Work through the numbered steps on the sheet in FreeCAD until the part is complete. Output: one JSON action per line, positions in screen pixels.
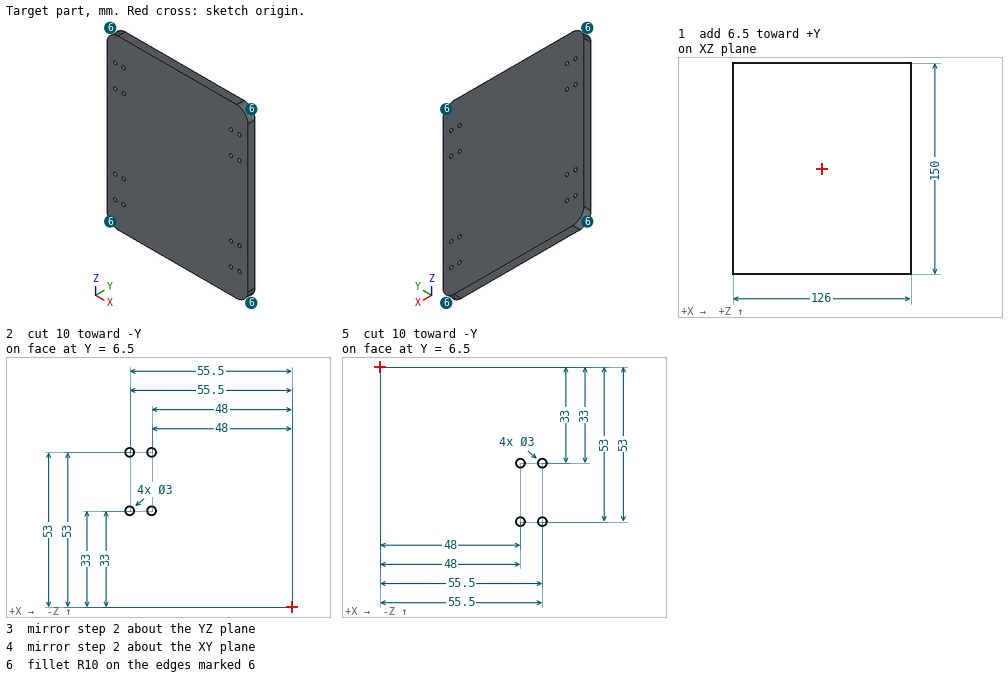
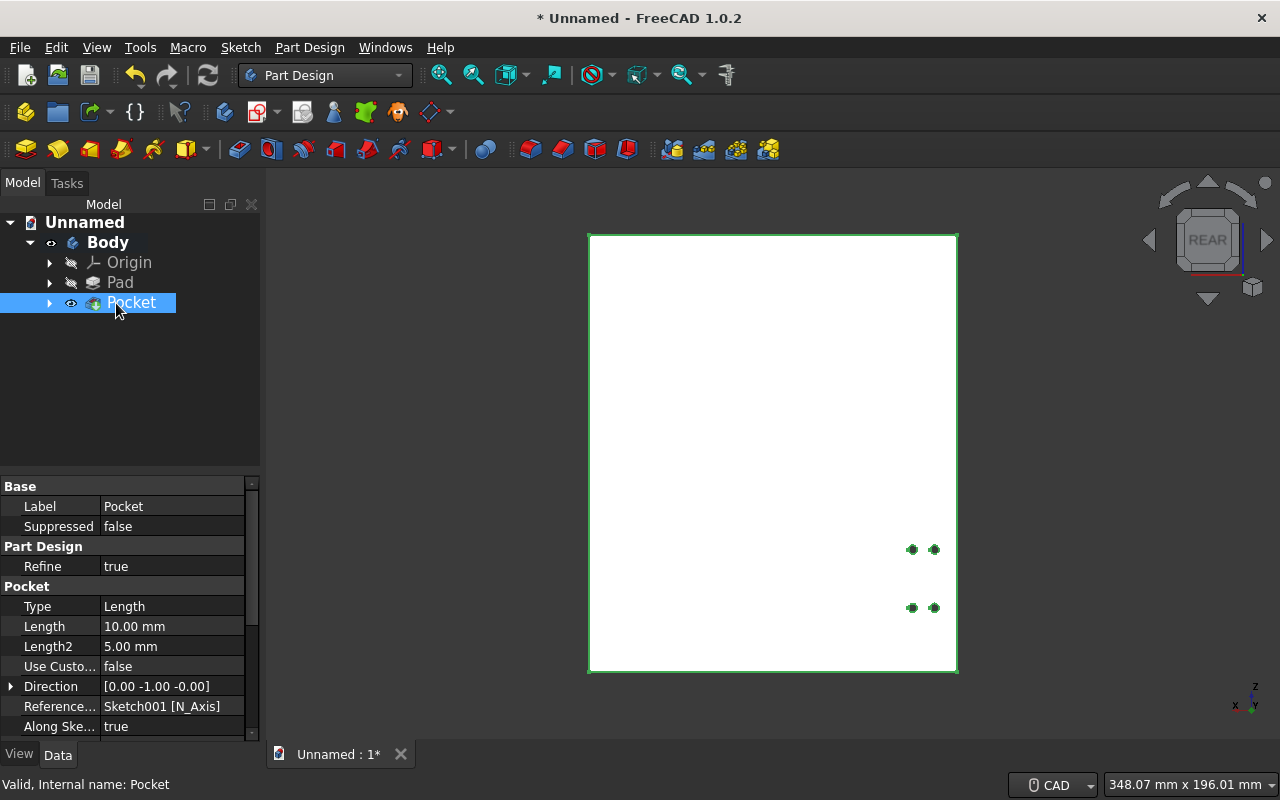
{"action": "left_click", "coordinate": [672, 150]}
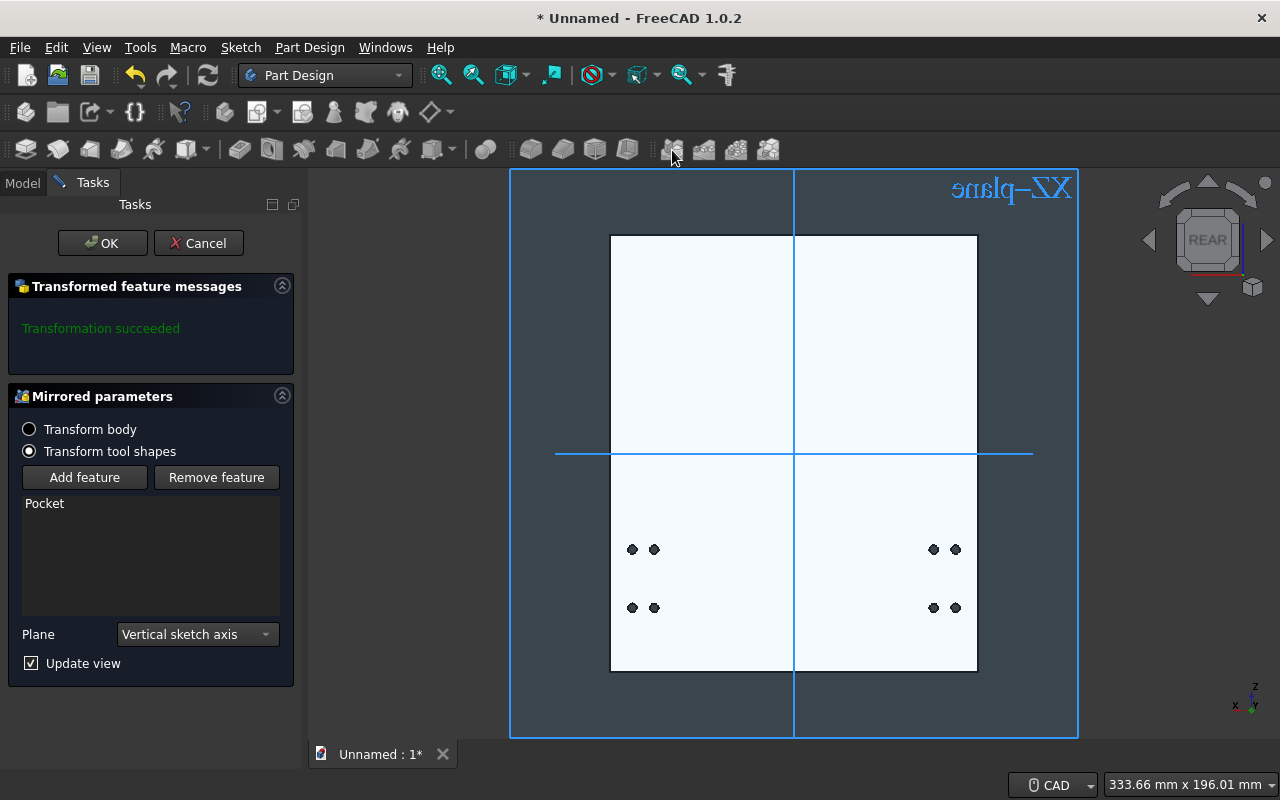
{"action": "left_click", "coordinate": [198, 634]}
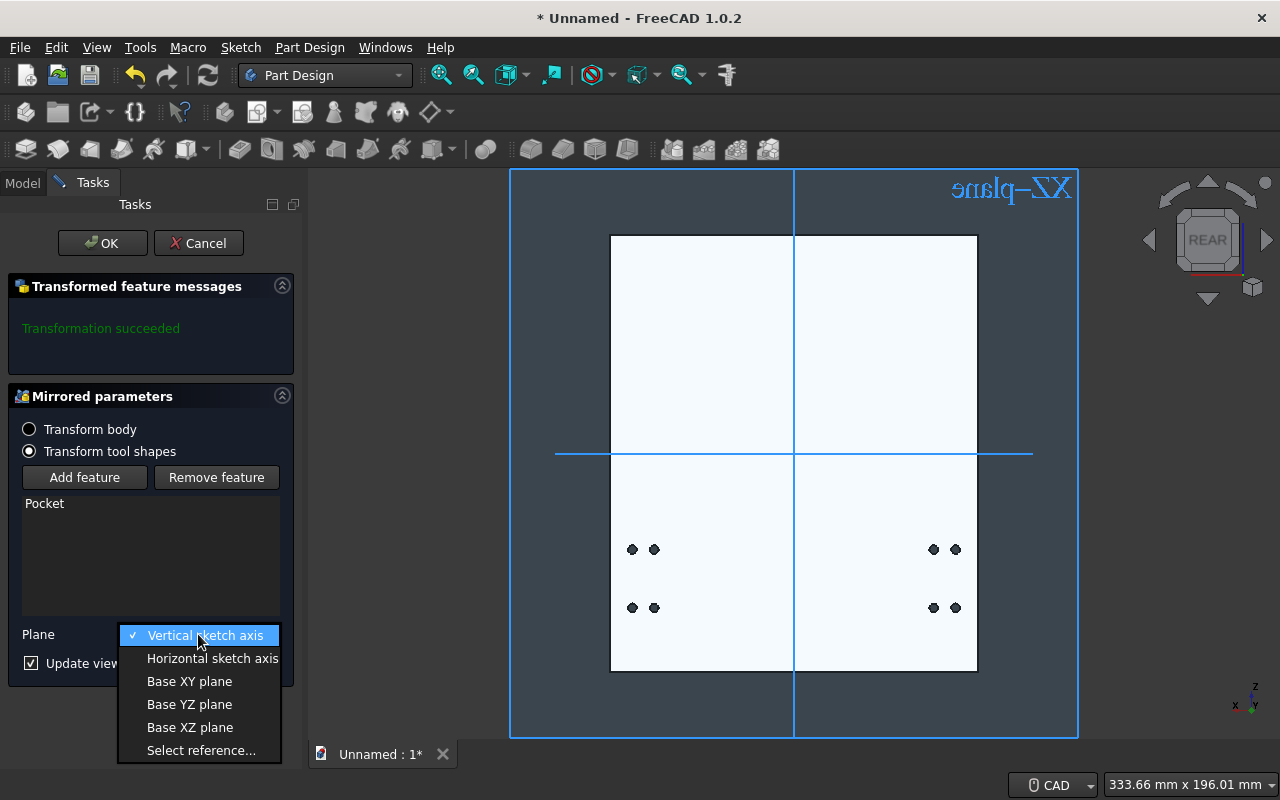
{"action": "left_click", "coordinate": [198, 704]}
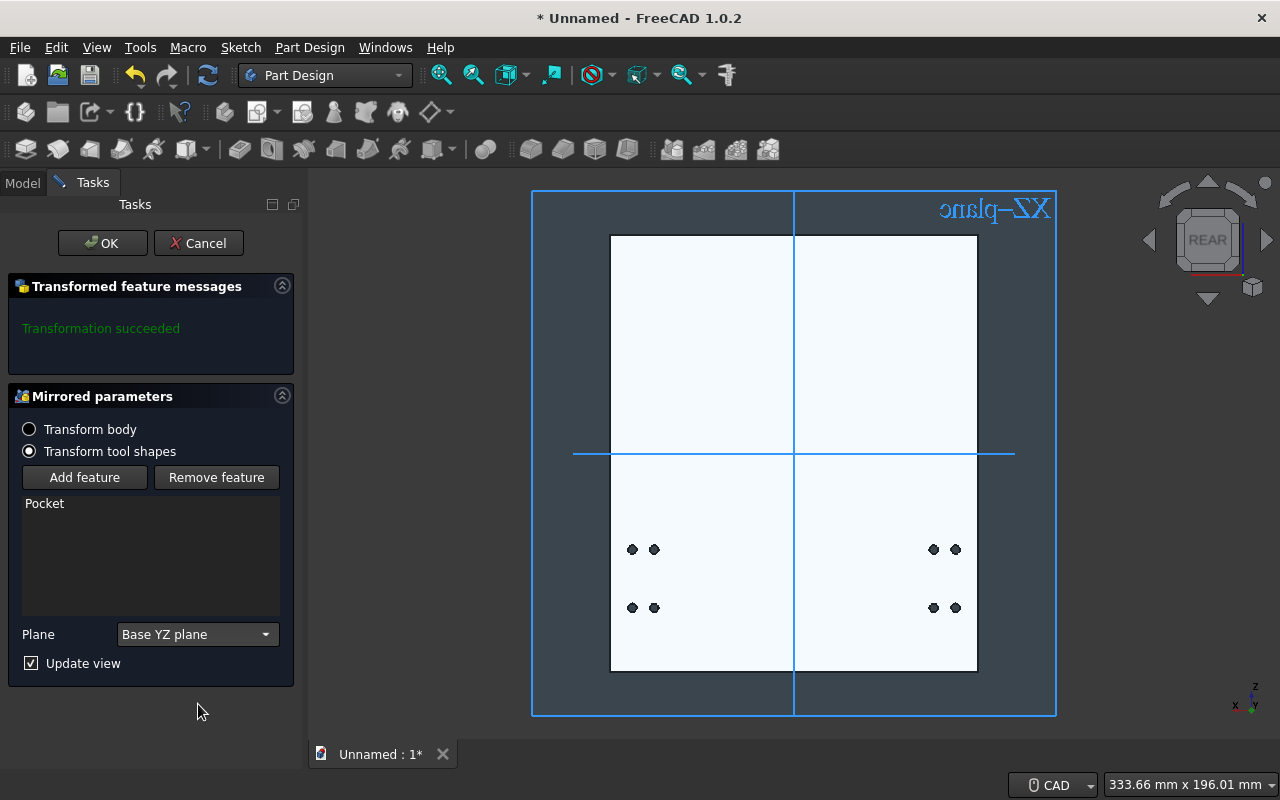
{"action": "left_click", "coordinate": [103, 243]}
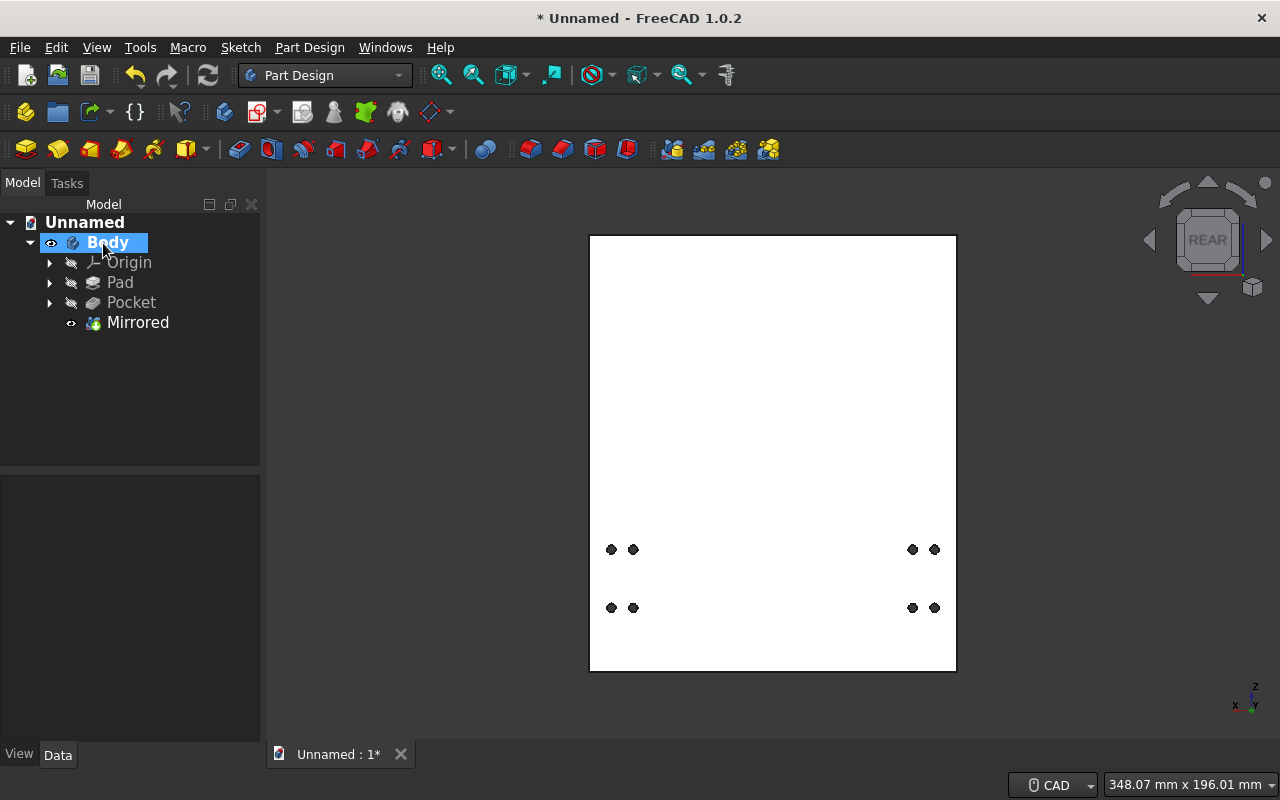
{"action": "left_click", "coordinate": [116, 303]}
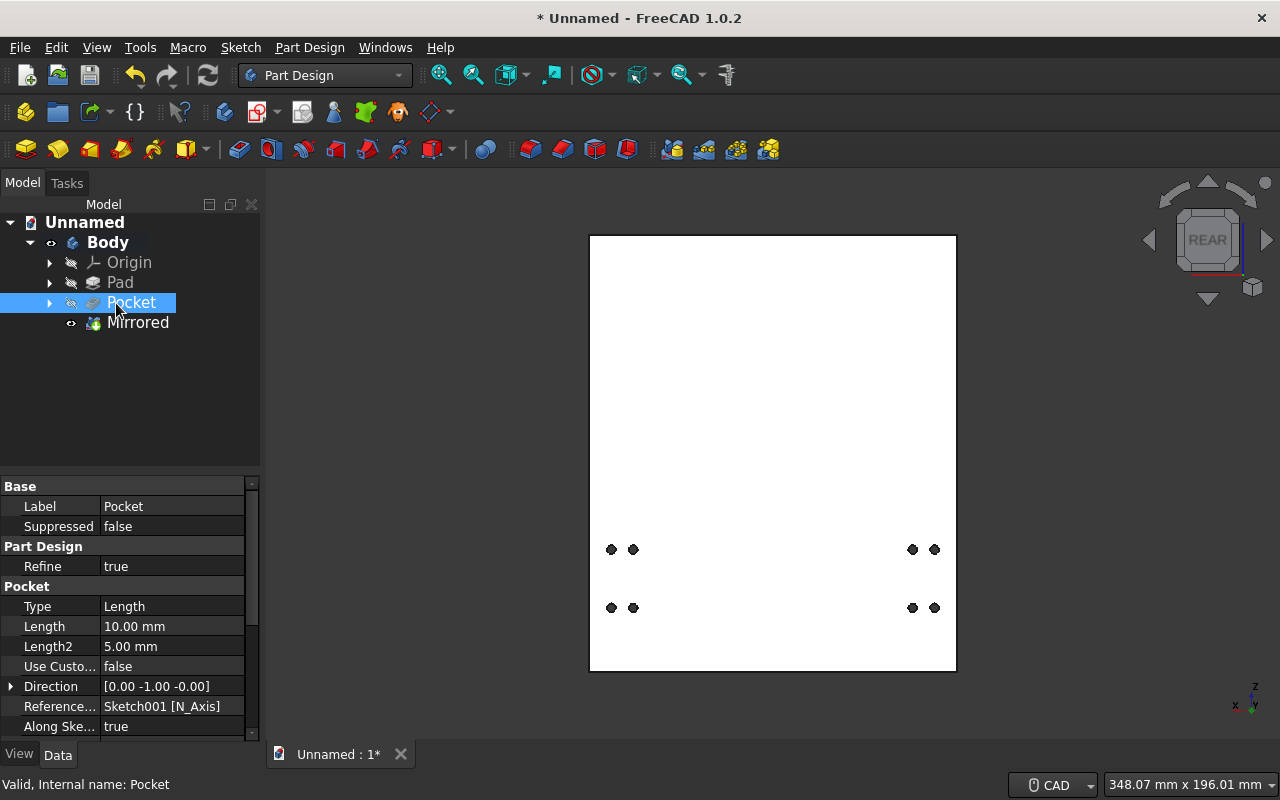
{"action": "left_click", "coordinate": [672, 150]}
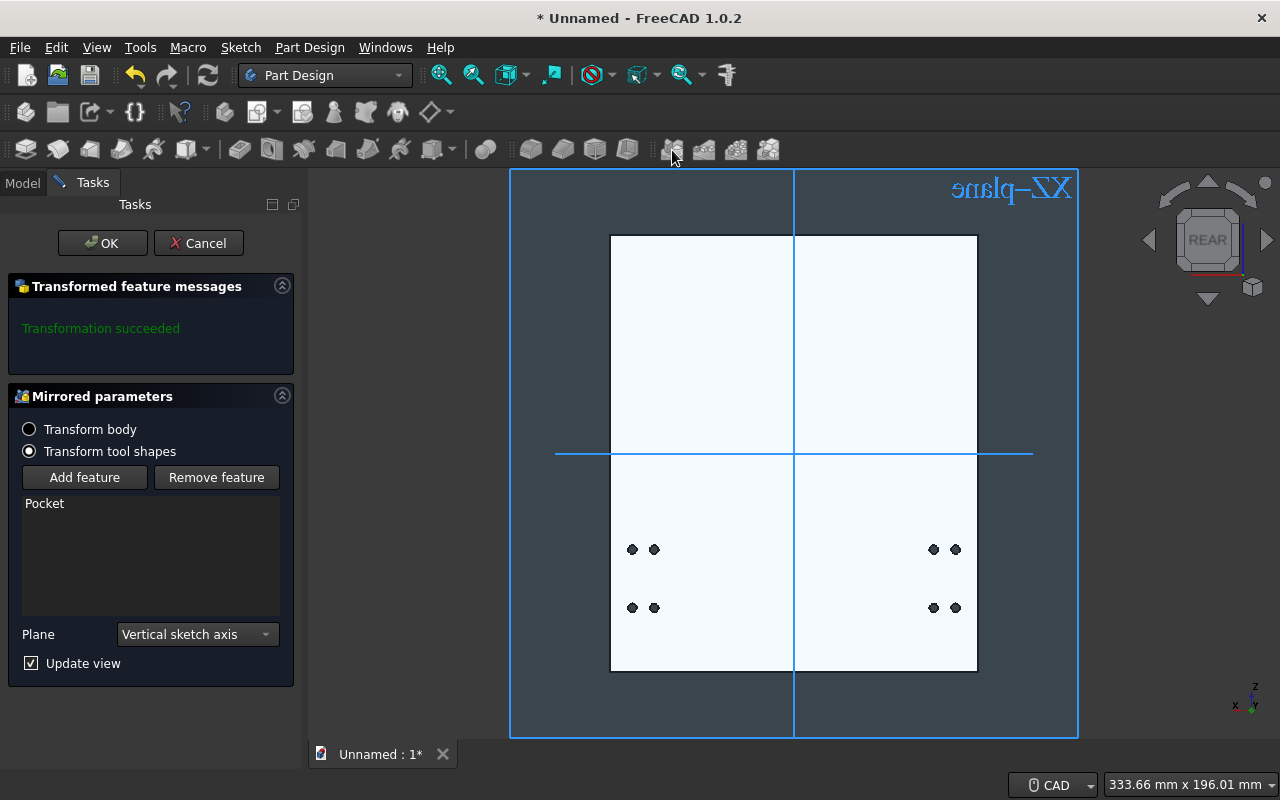
{"action": "left_click", "coordinate": [198, 634]}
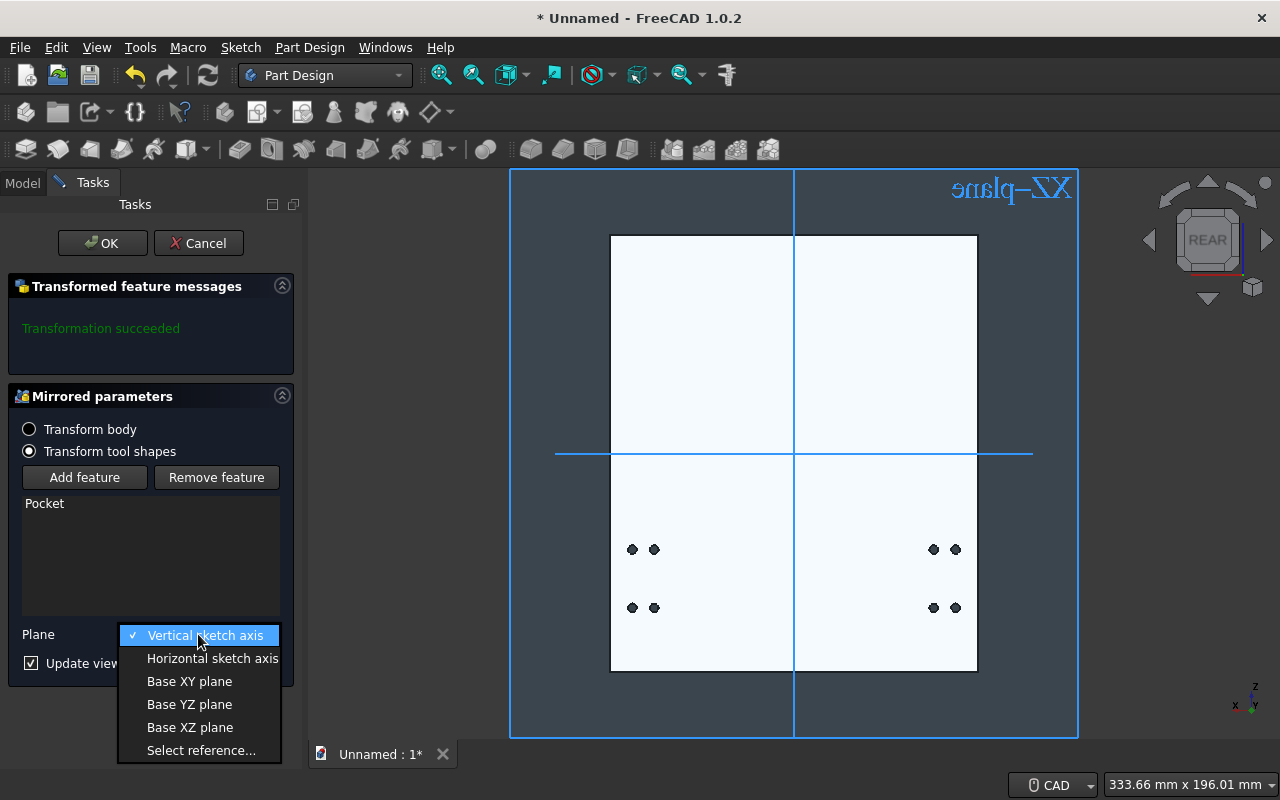
{"action": "left_click", "coordinate": [198, 682]}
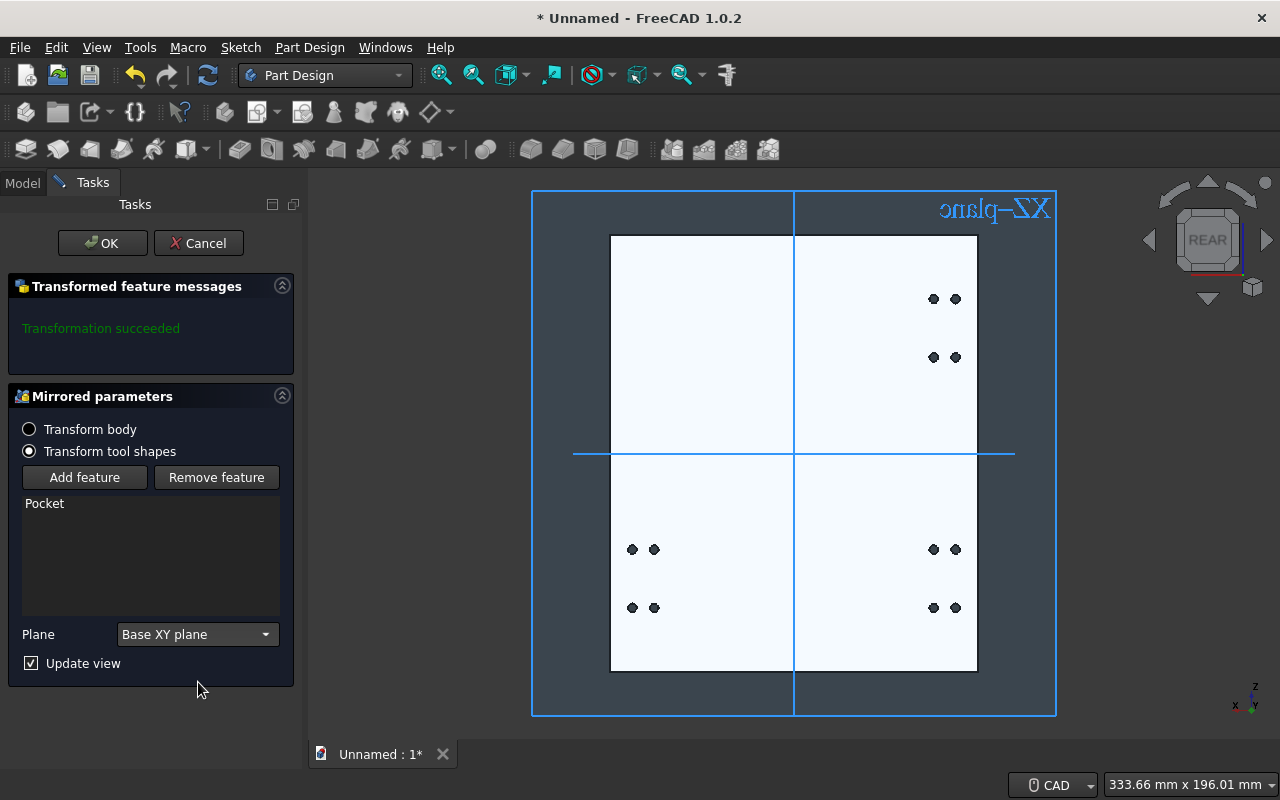
{"action": "left_click", "coordinate": [103, 243]}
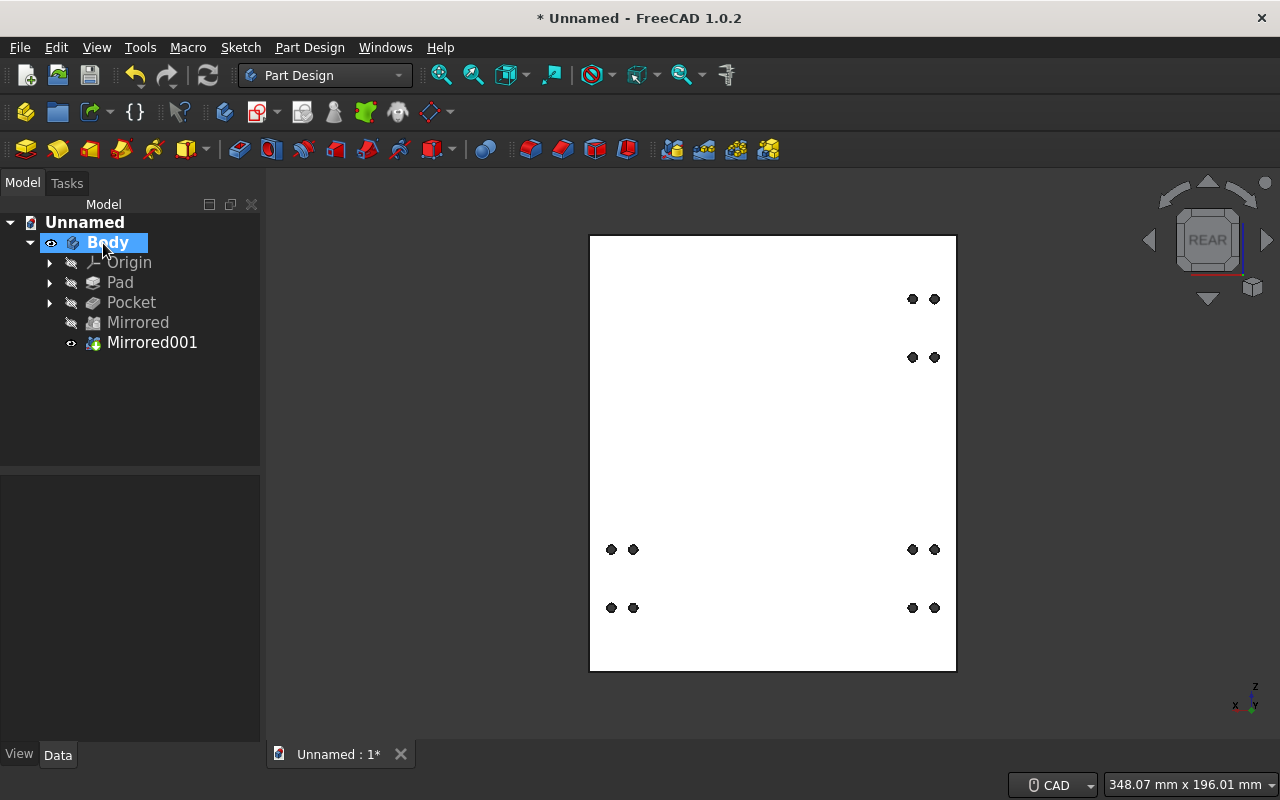
{"action": "left_click", "coordinate": [773, 452]}